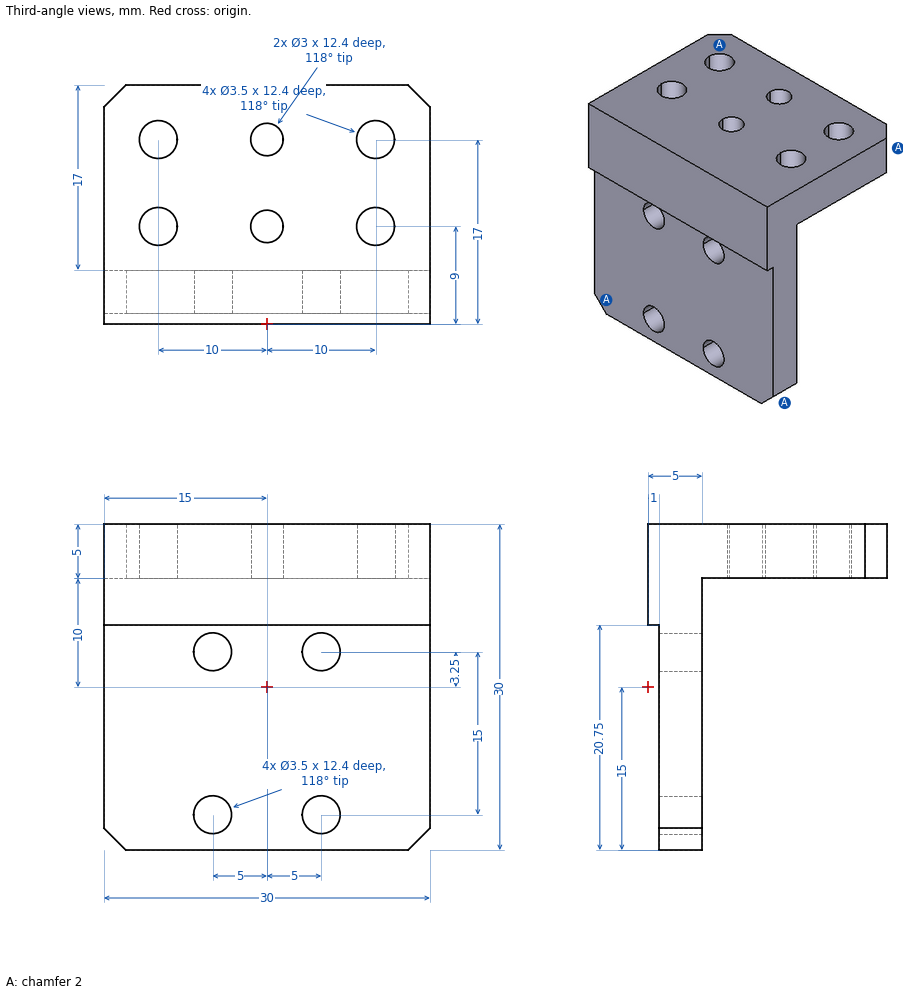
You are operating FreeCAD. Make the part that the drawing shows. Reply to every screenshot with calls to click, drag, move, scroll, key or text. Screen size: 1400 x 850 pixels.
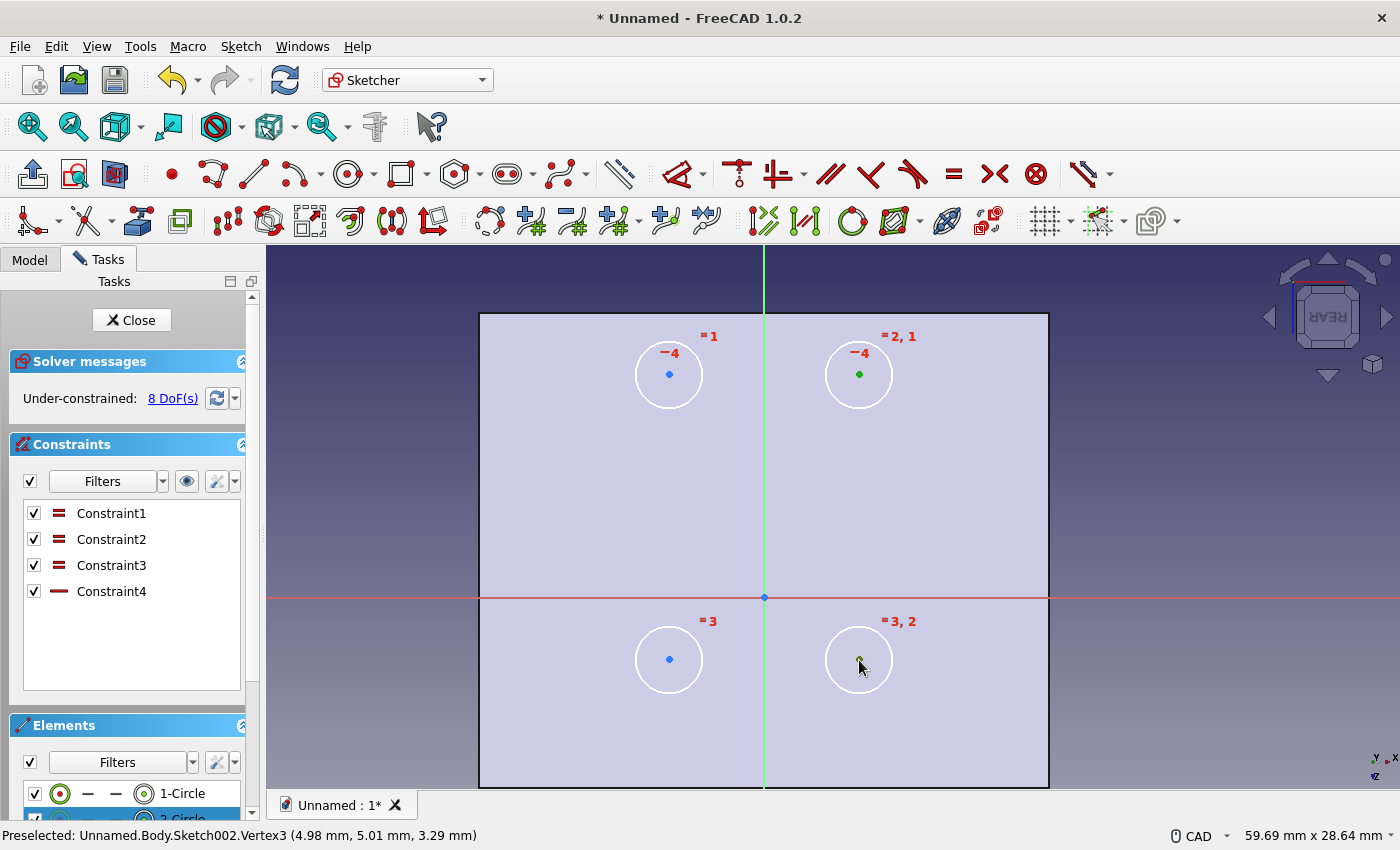
key(v)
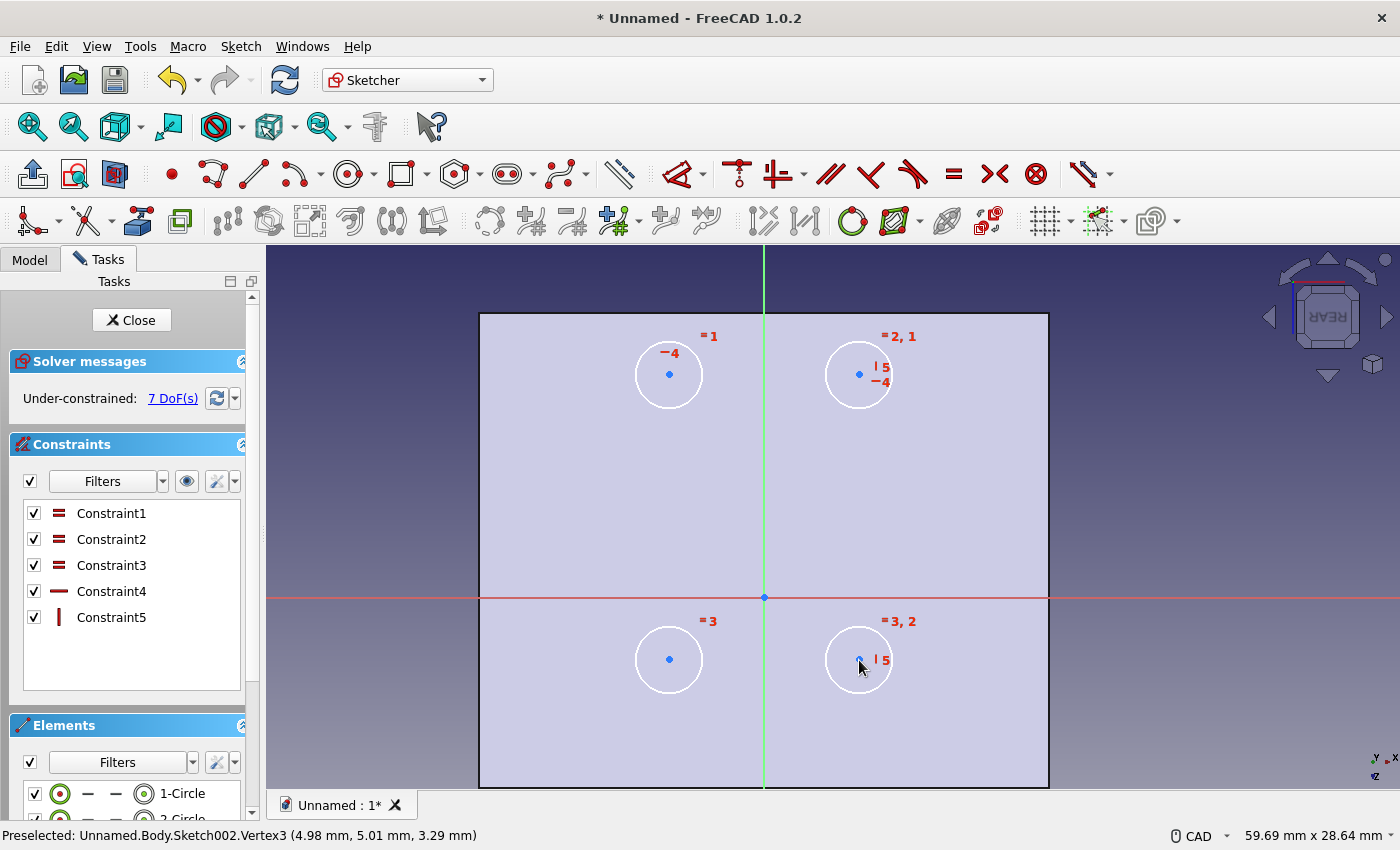
click(669, 375)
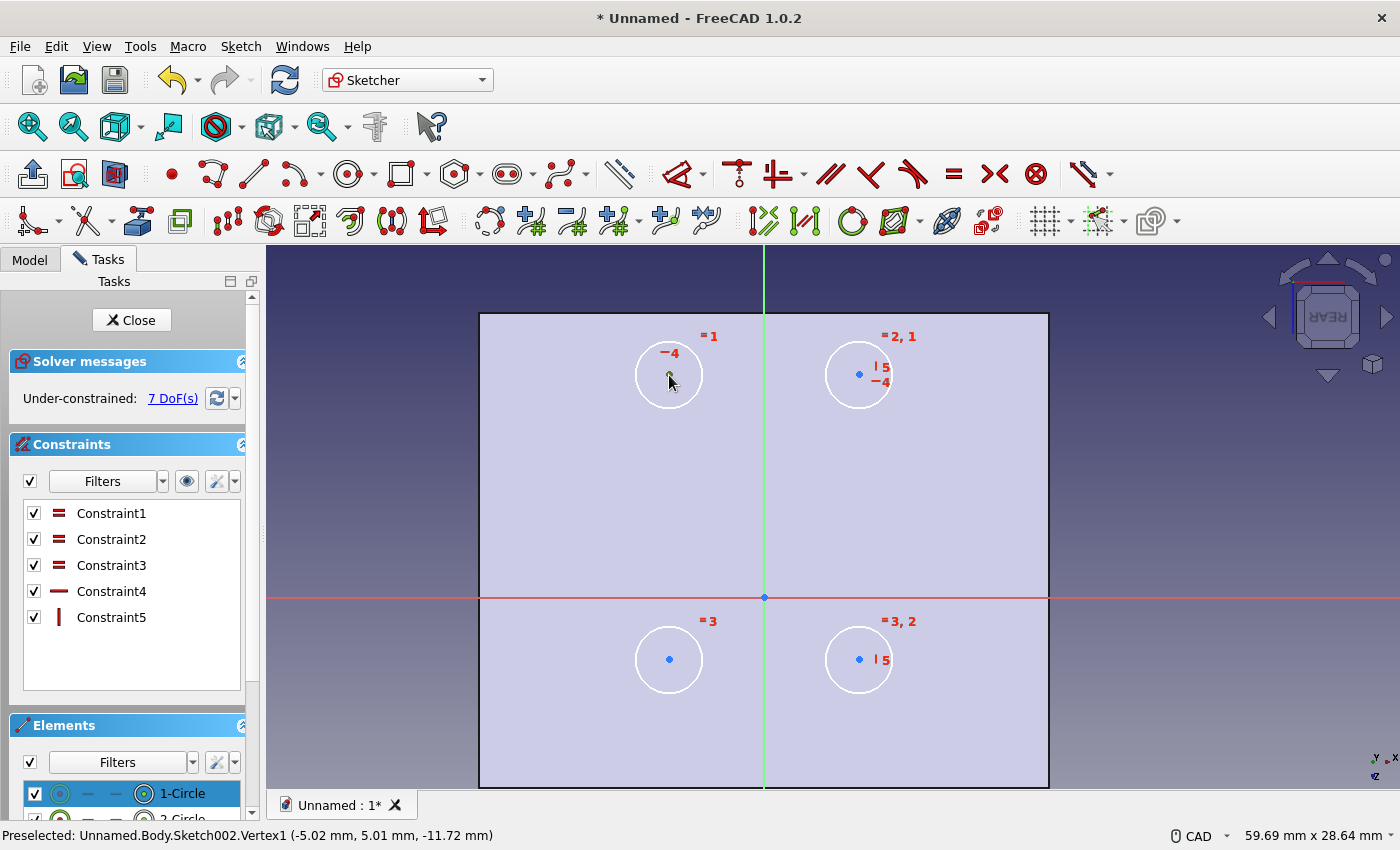
click(669, 660)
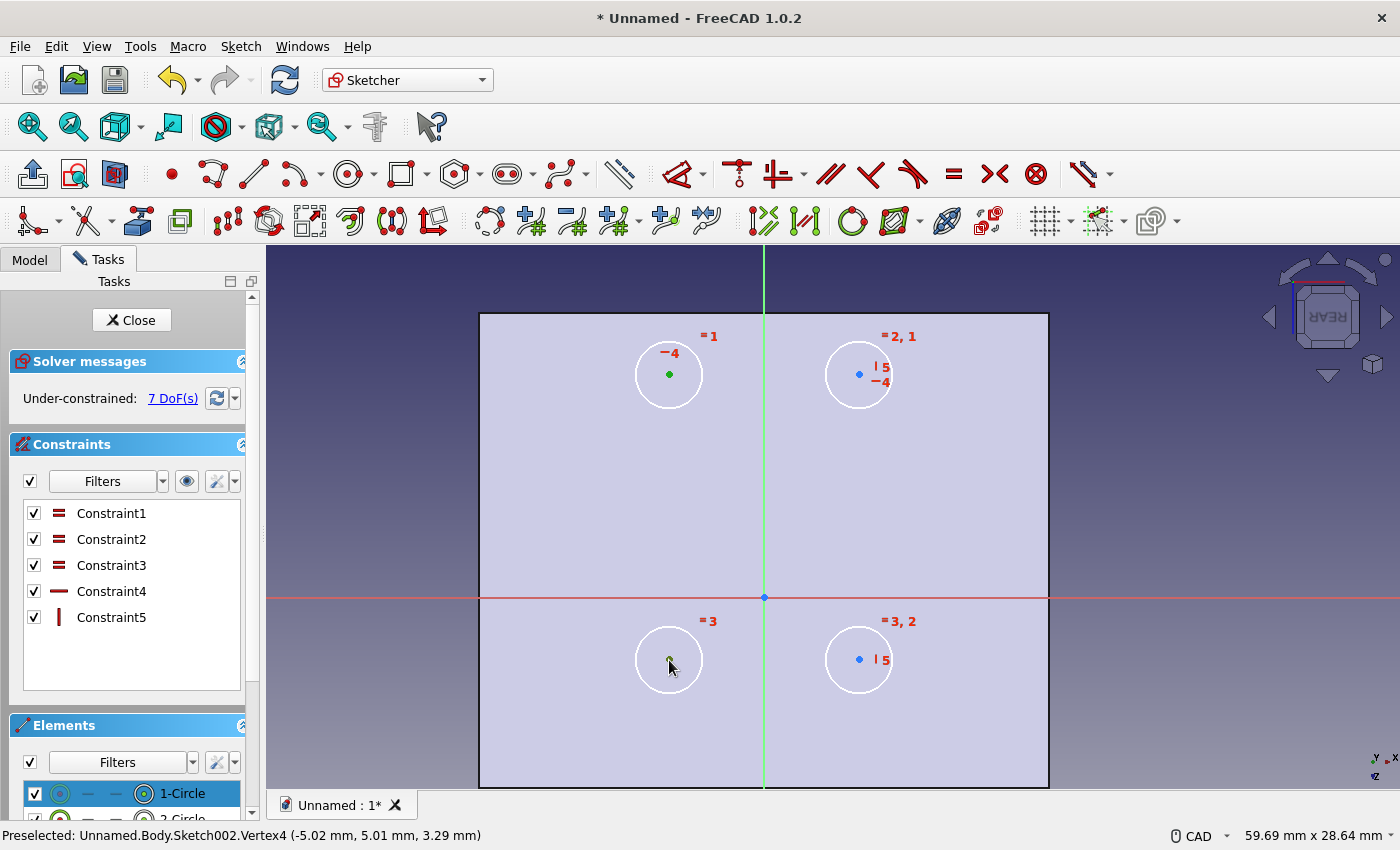
key(v)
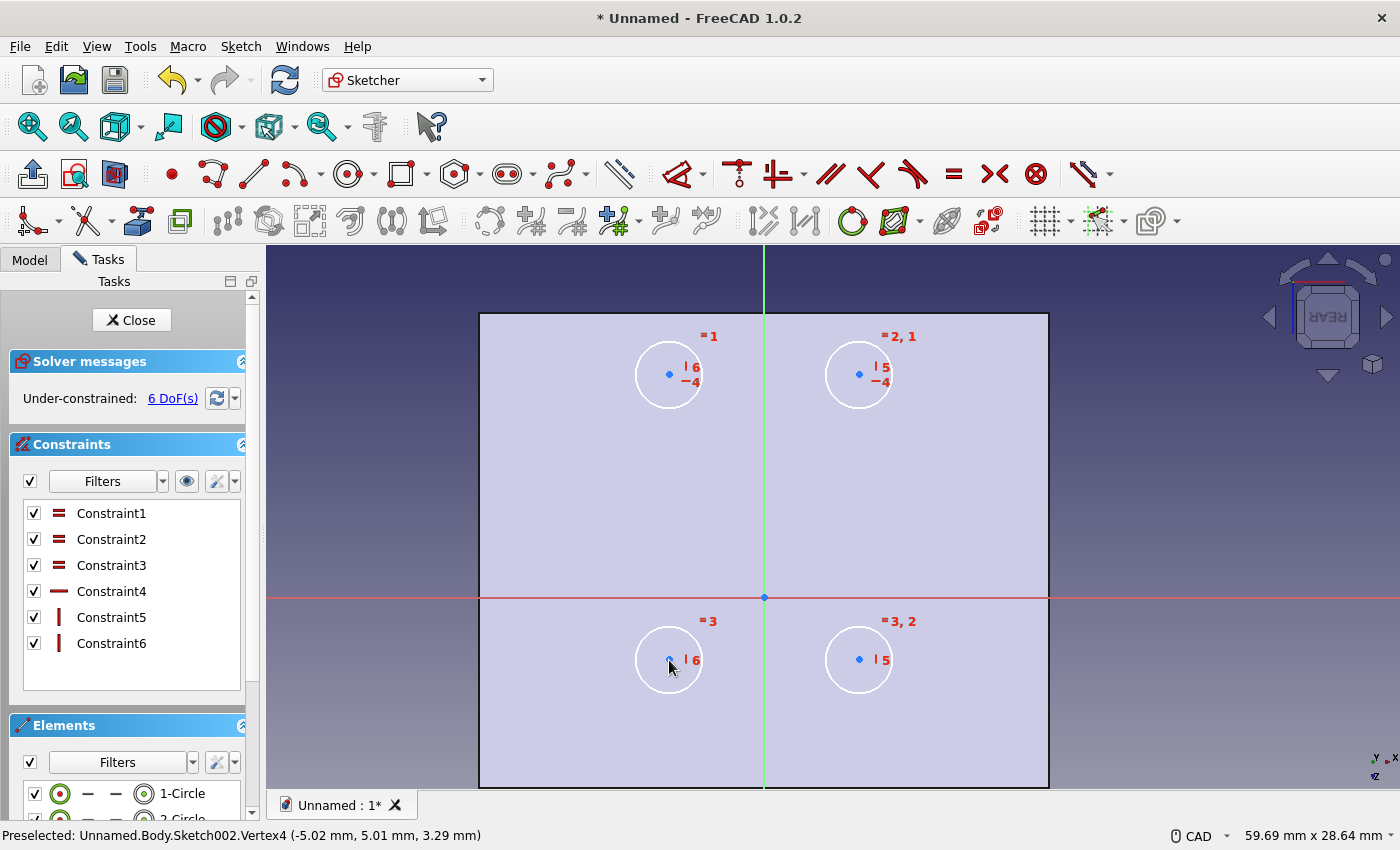
click(859, 660)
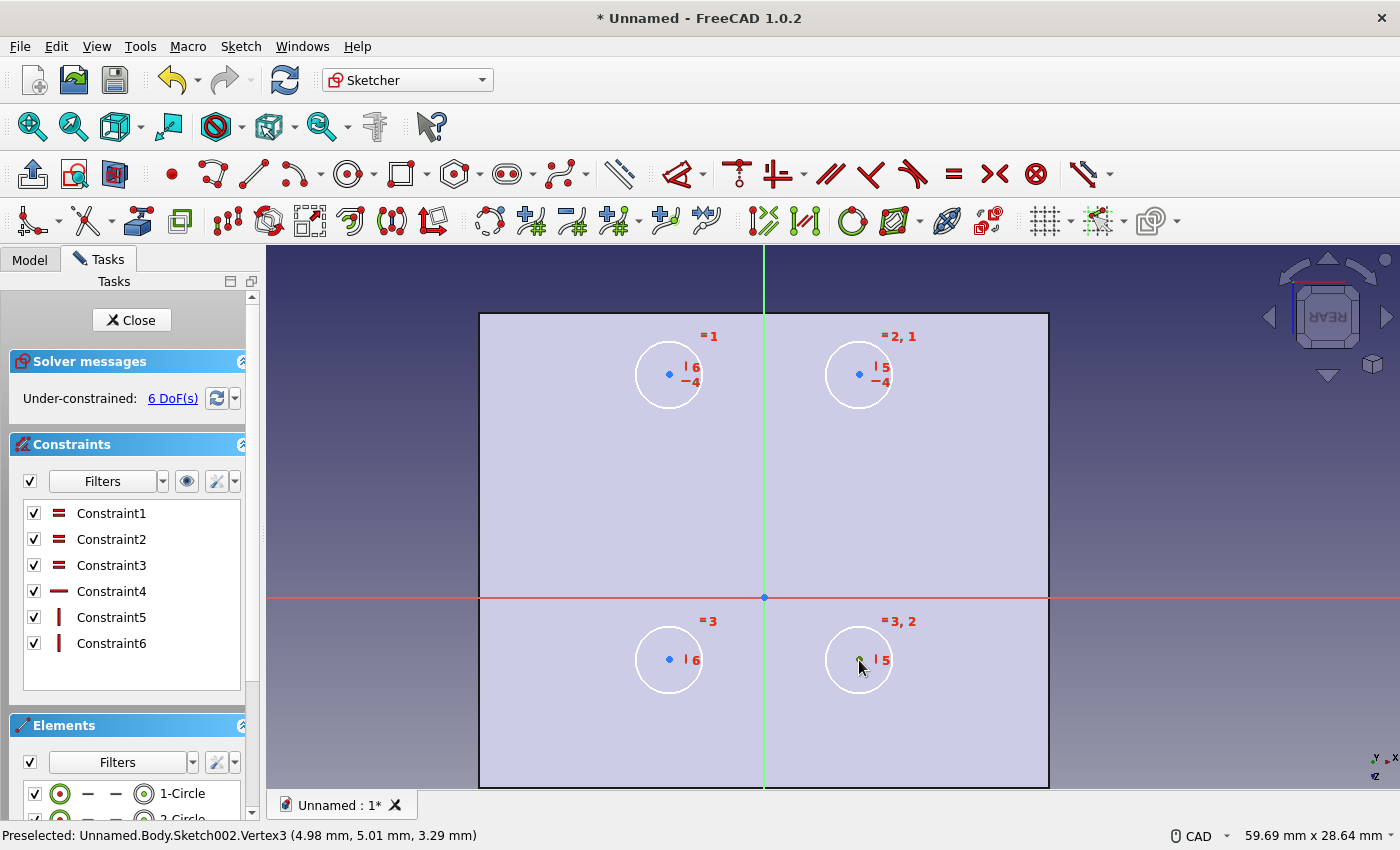
click(669, 660)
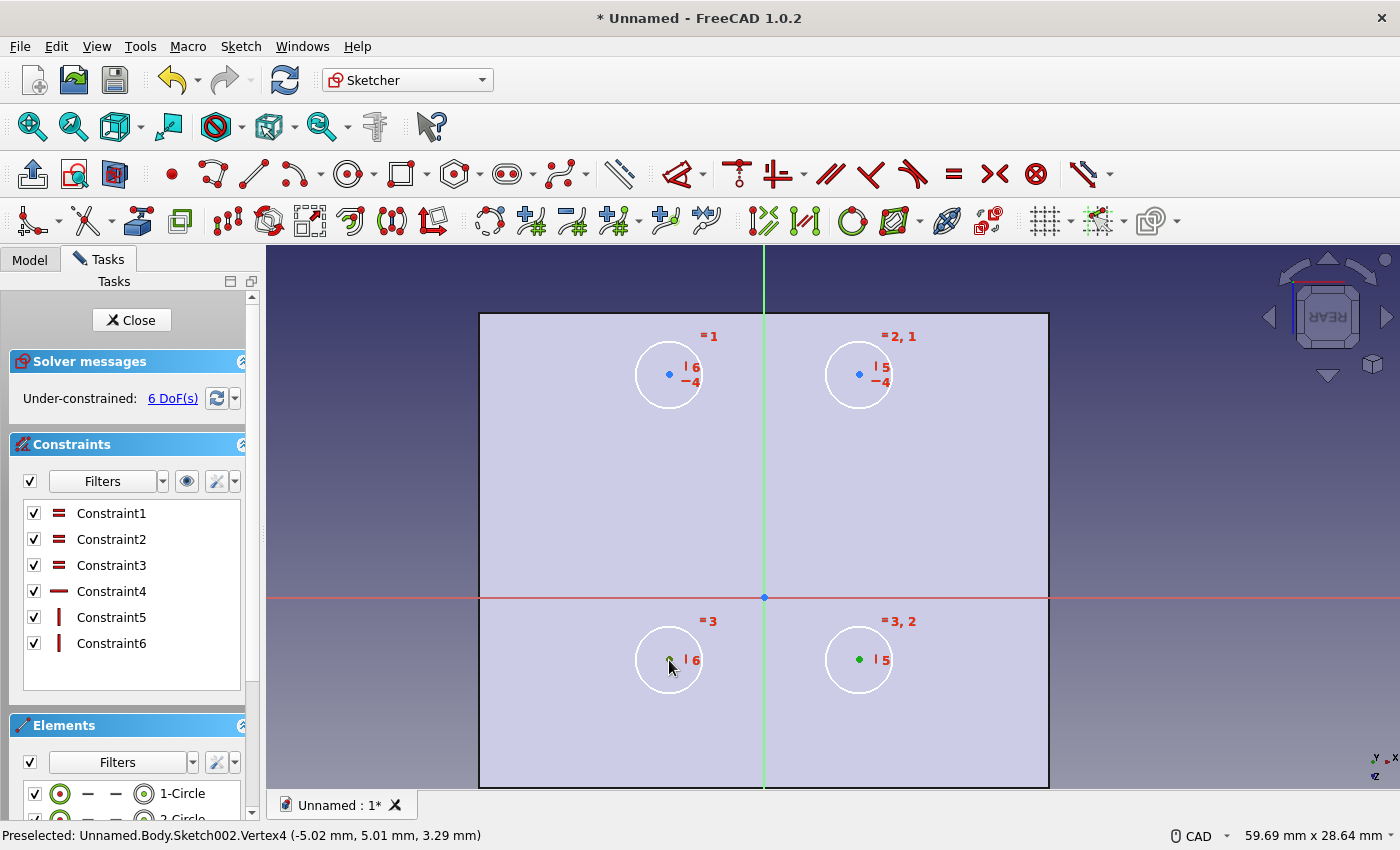
key(h)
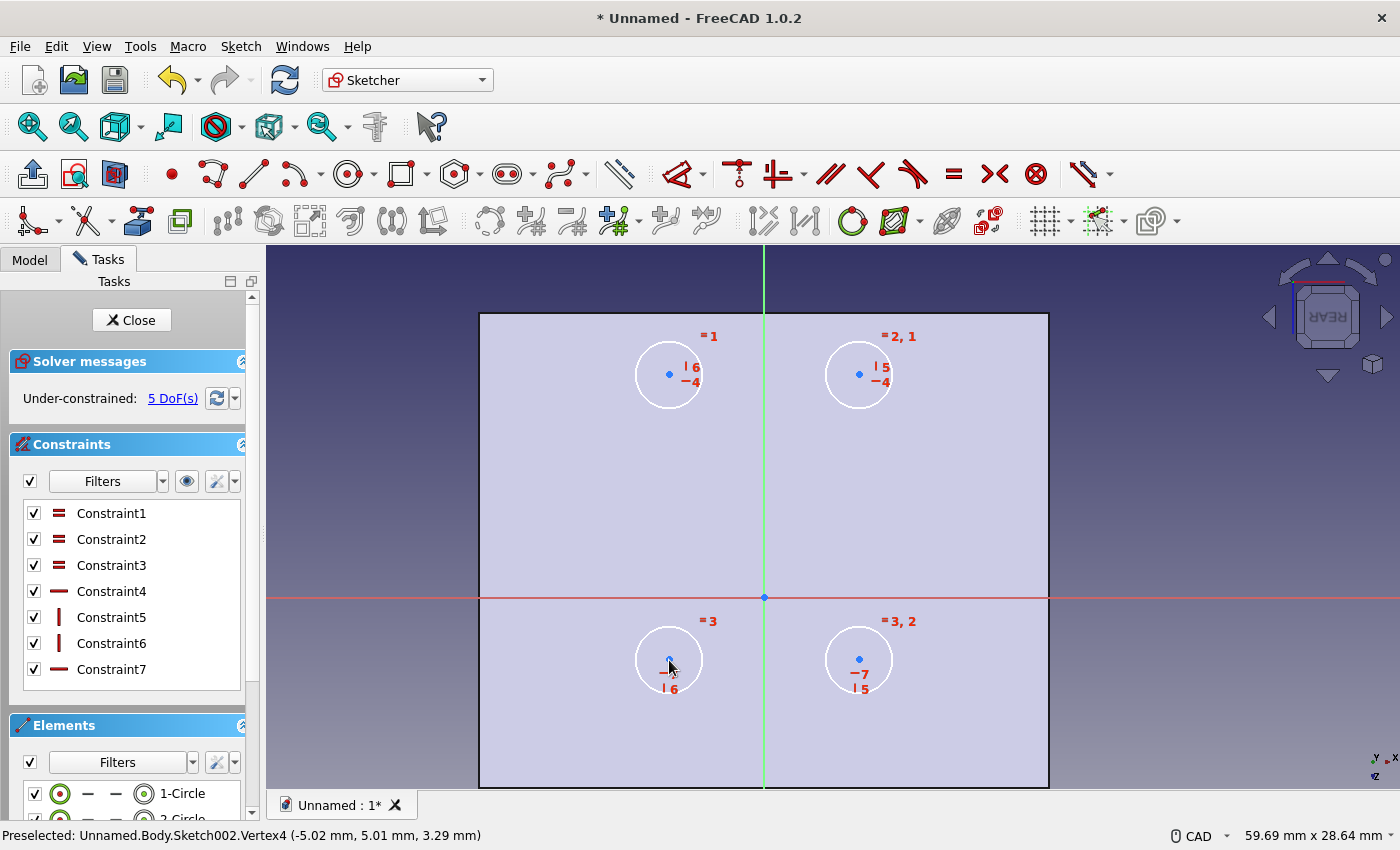
key(d)